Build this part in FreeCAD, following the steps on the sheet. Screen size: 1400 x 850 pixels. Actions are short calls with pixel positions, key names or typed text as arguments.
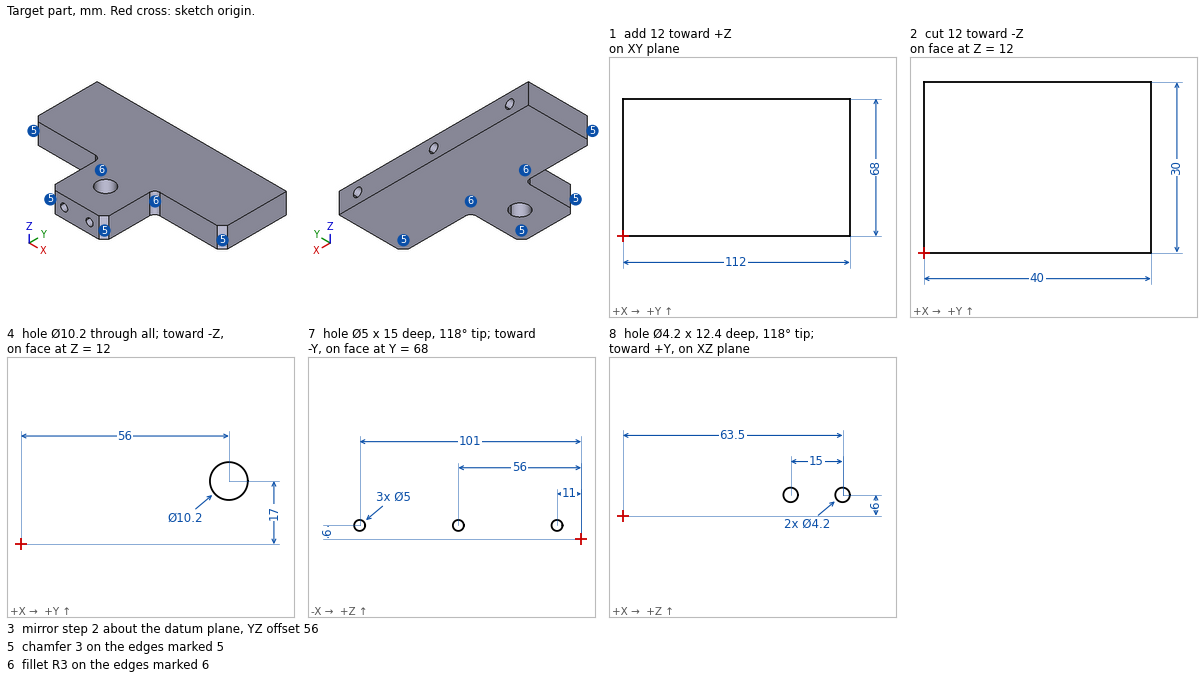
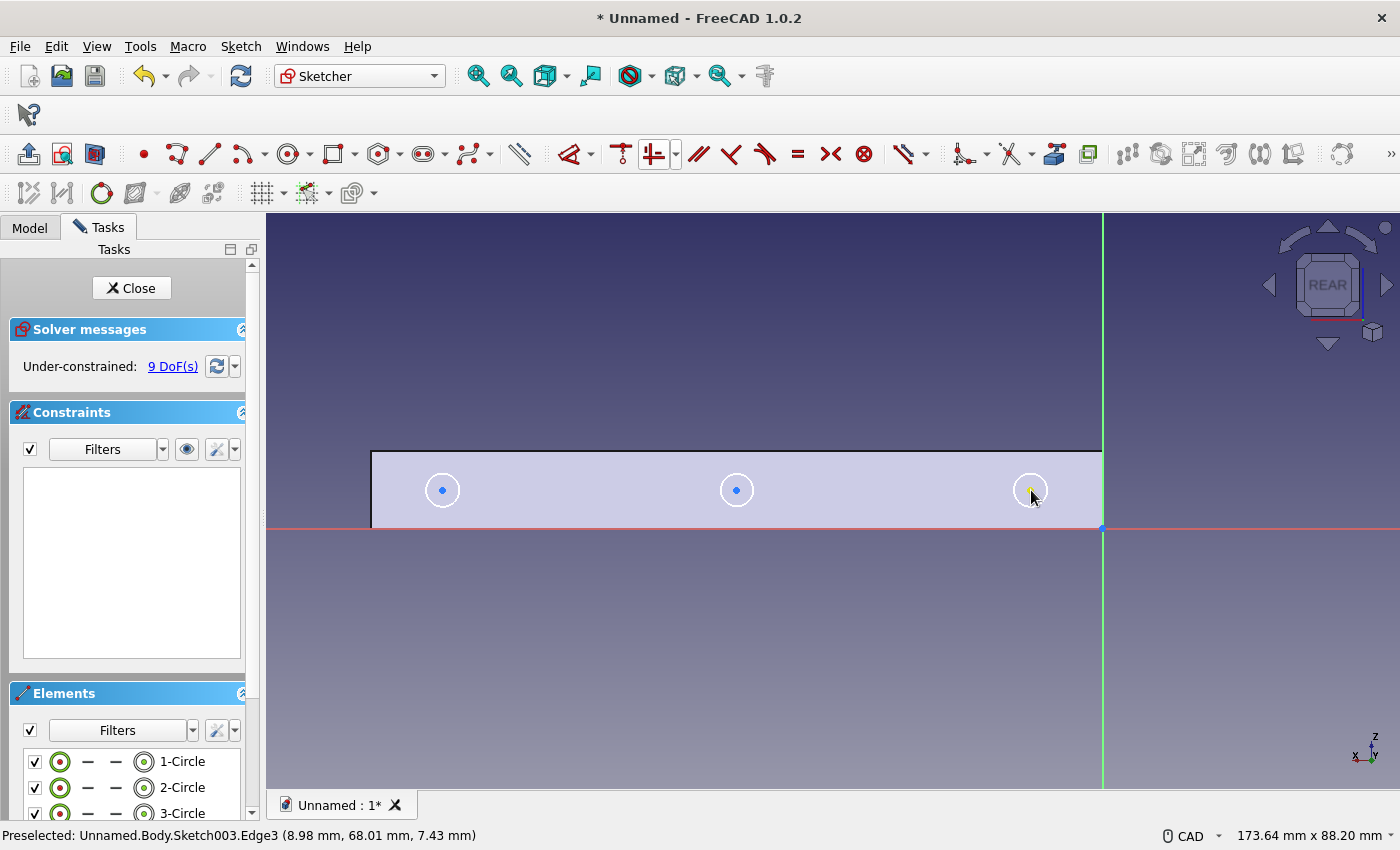
click(454, 478)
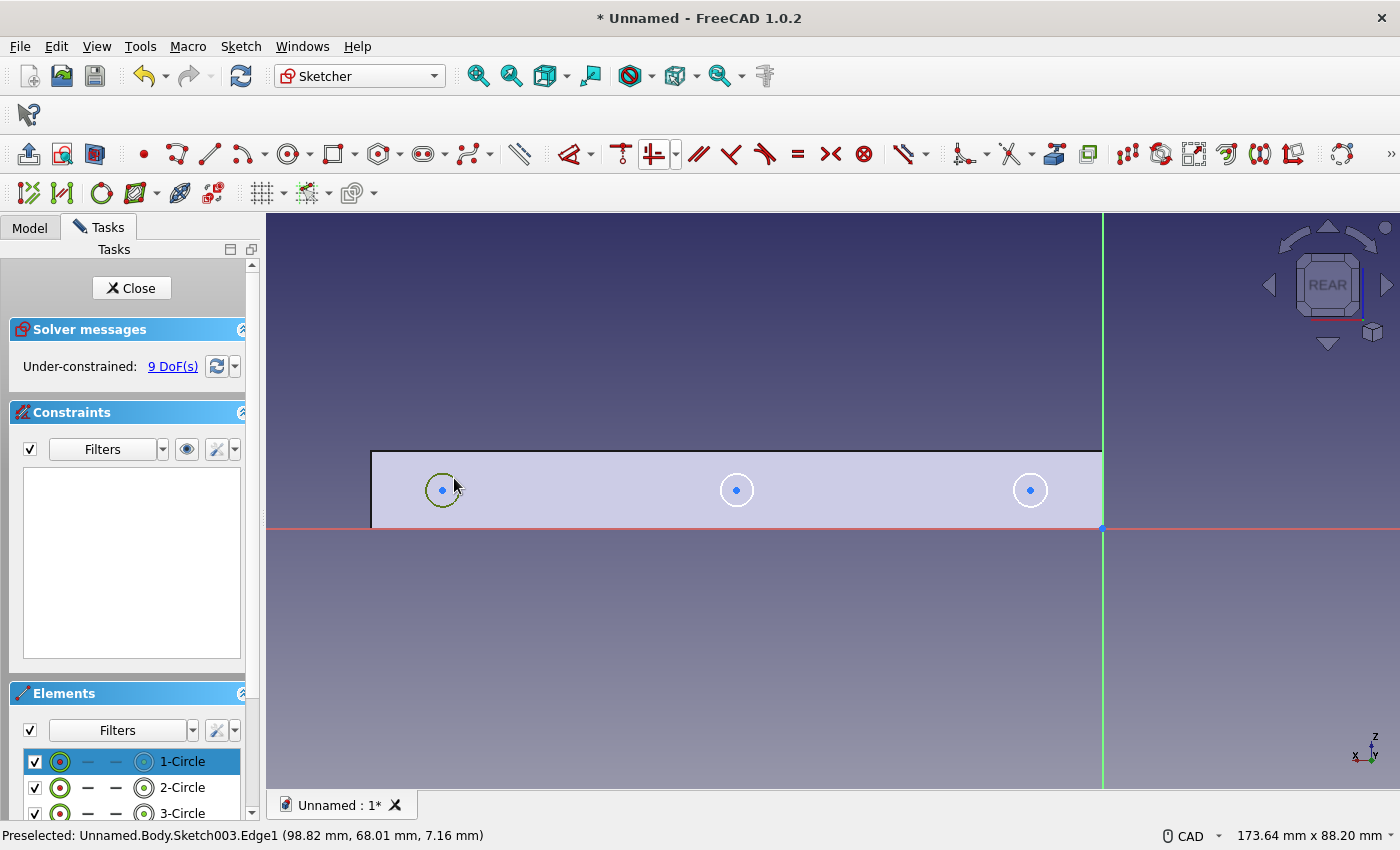
click(748, 479)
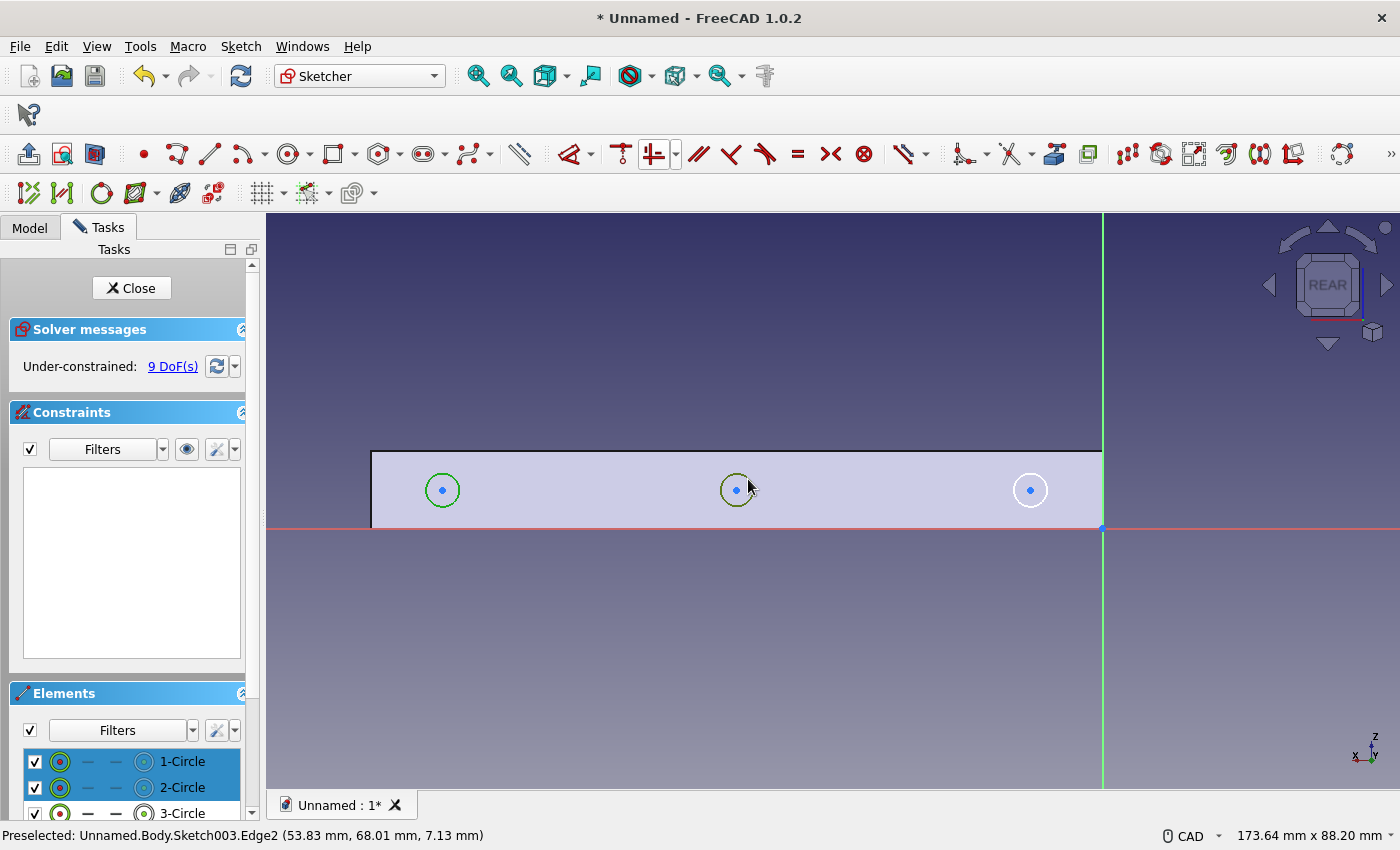
click(1042, 478)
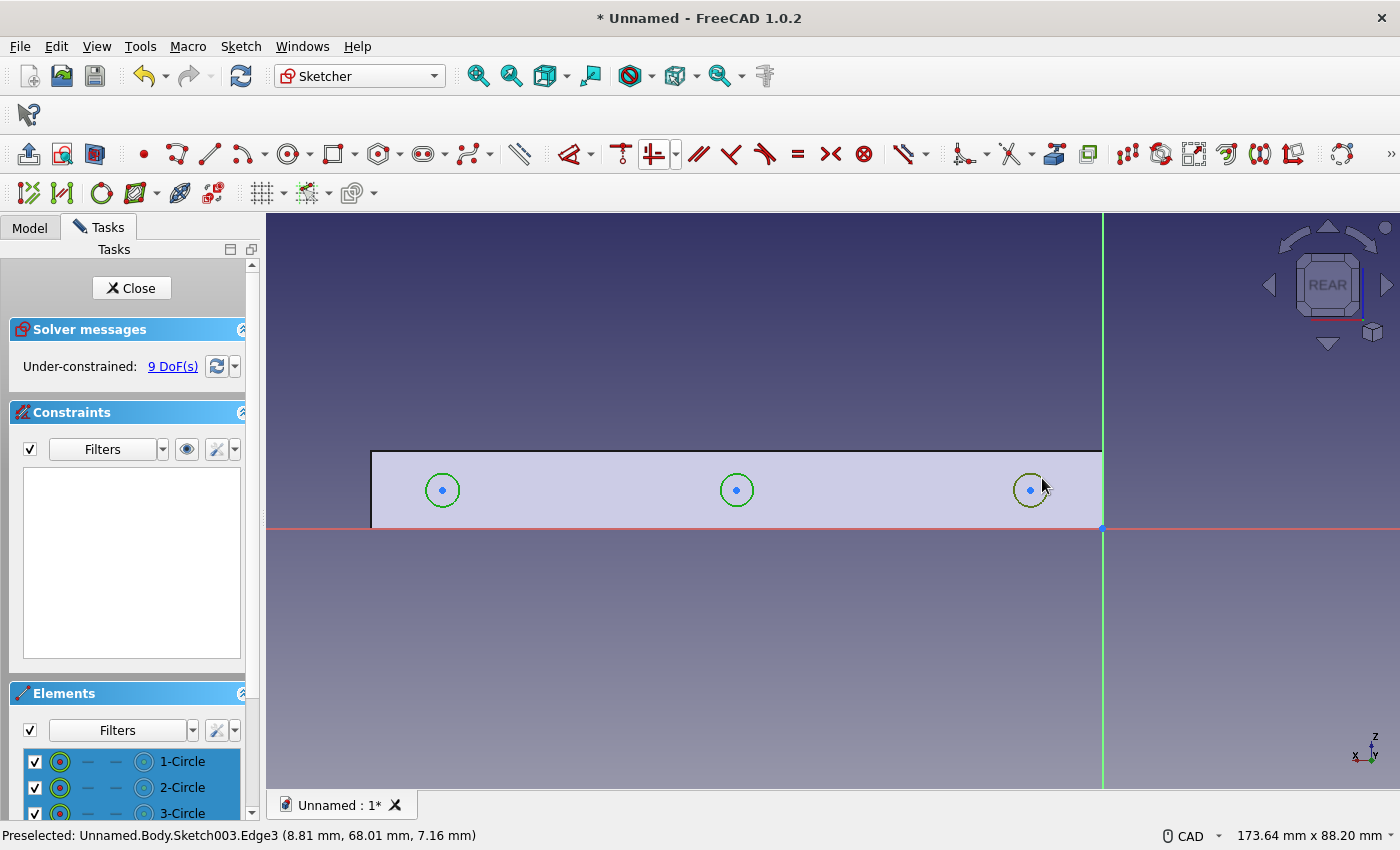
click(798, 154)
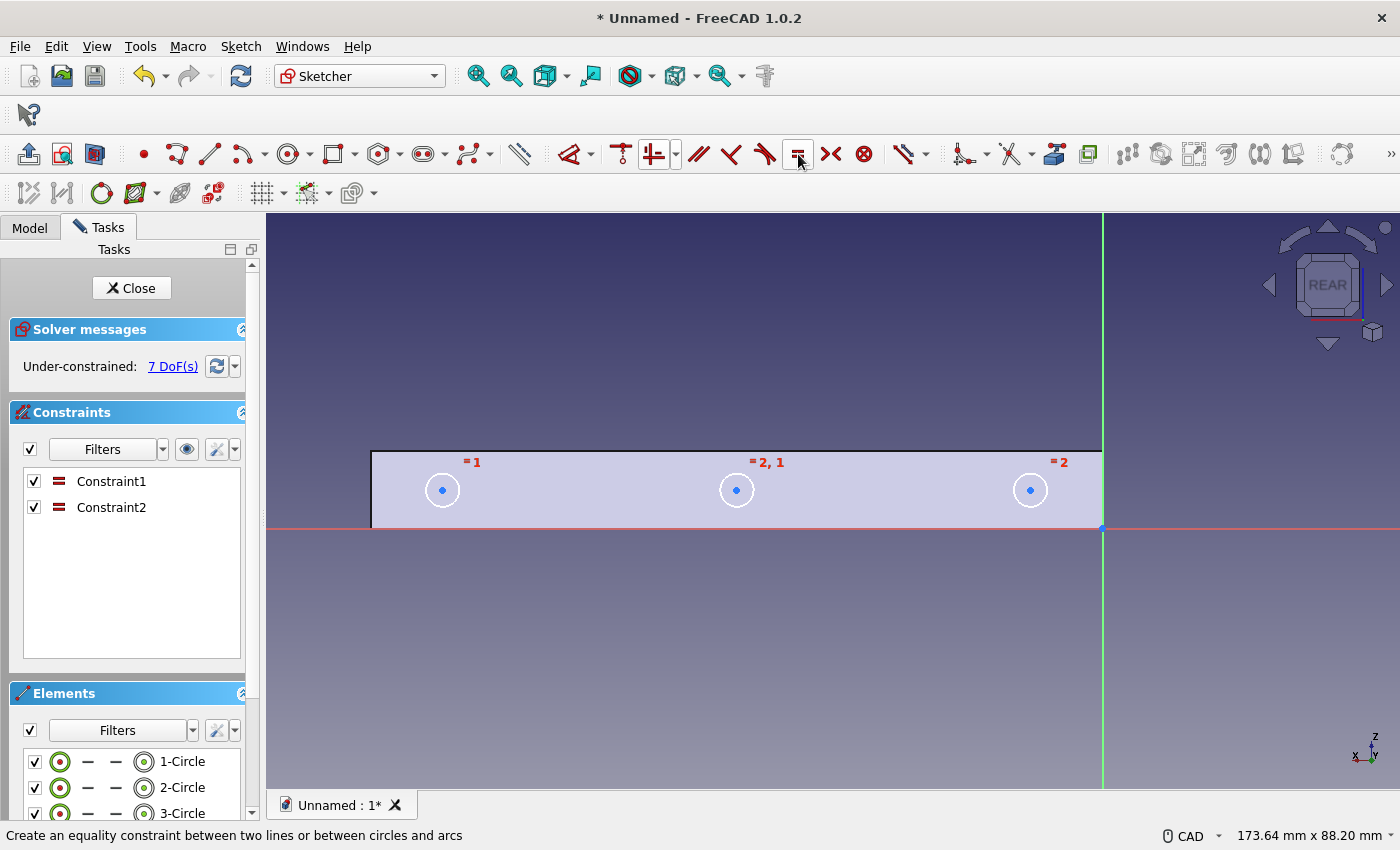
click(443, 490)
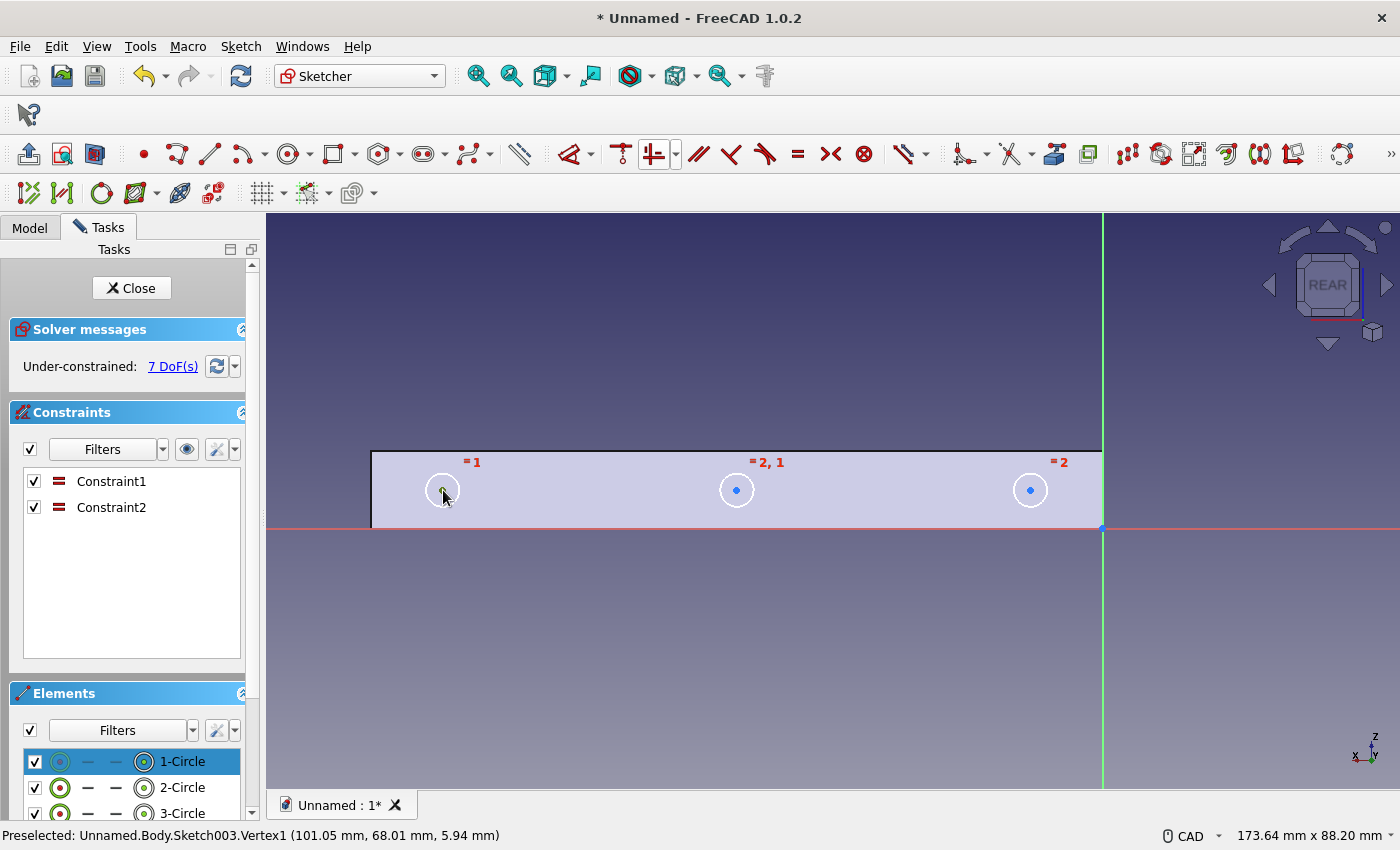
click(737, 490)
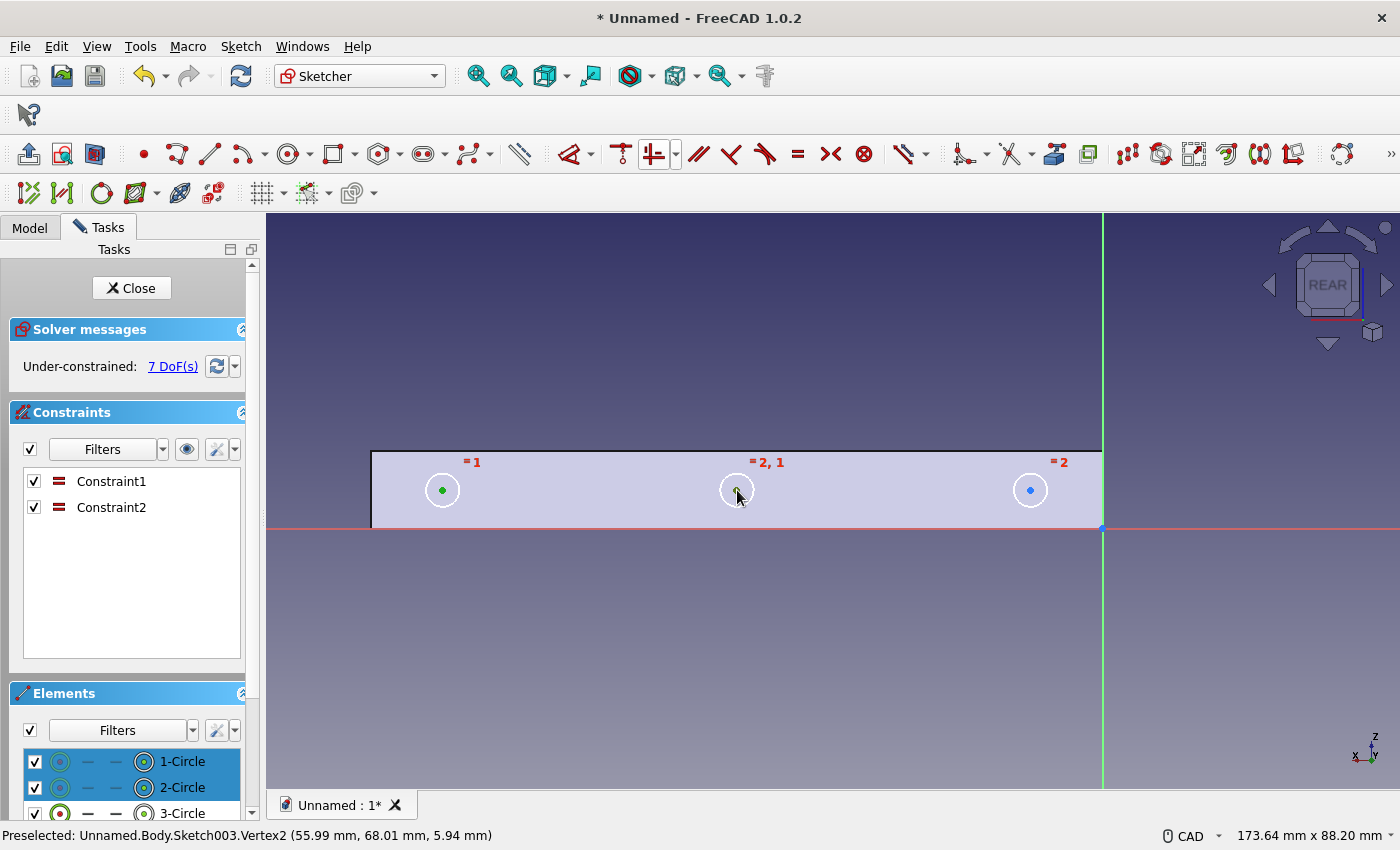
click(676, 154)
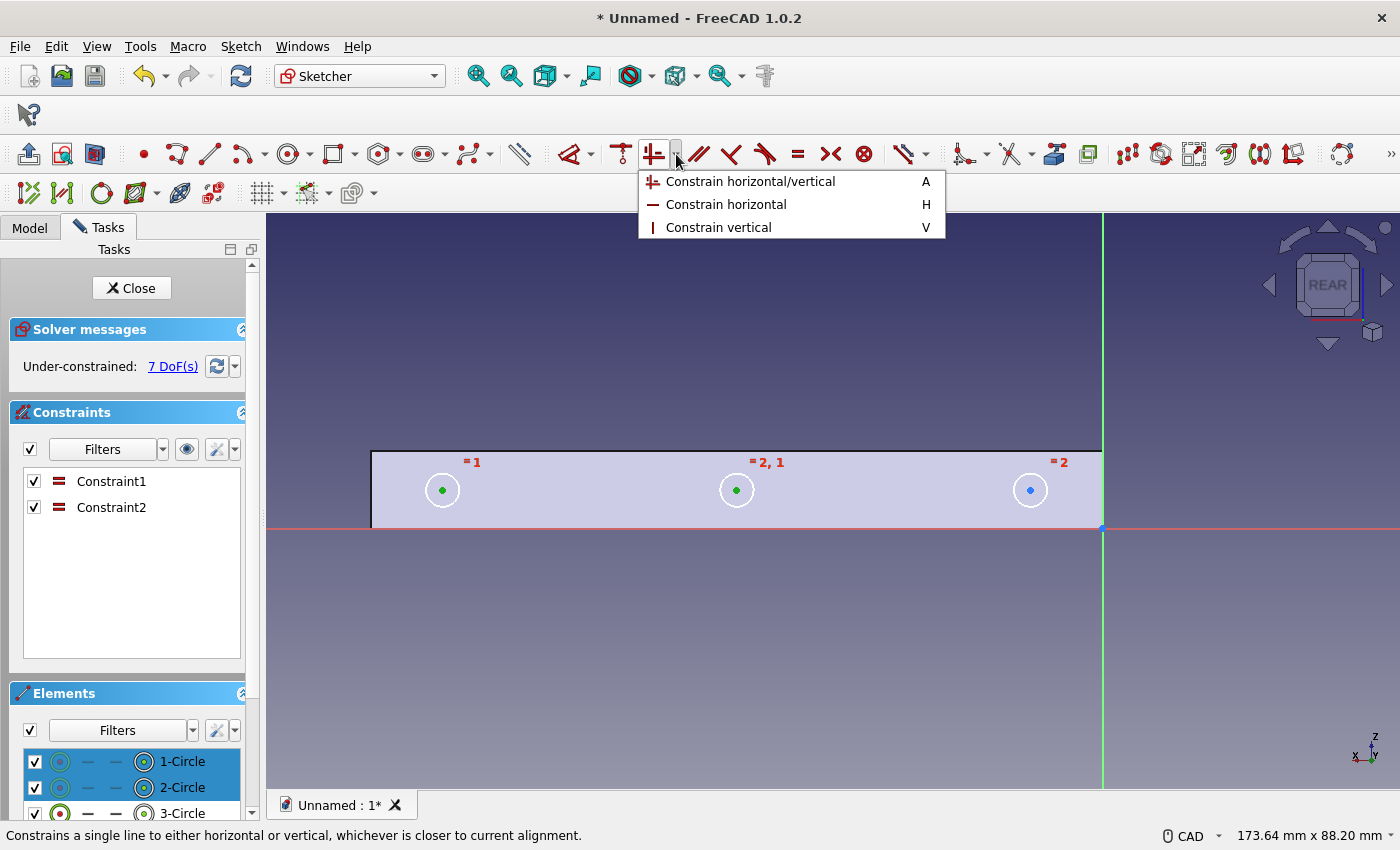
click(792, 204)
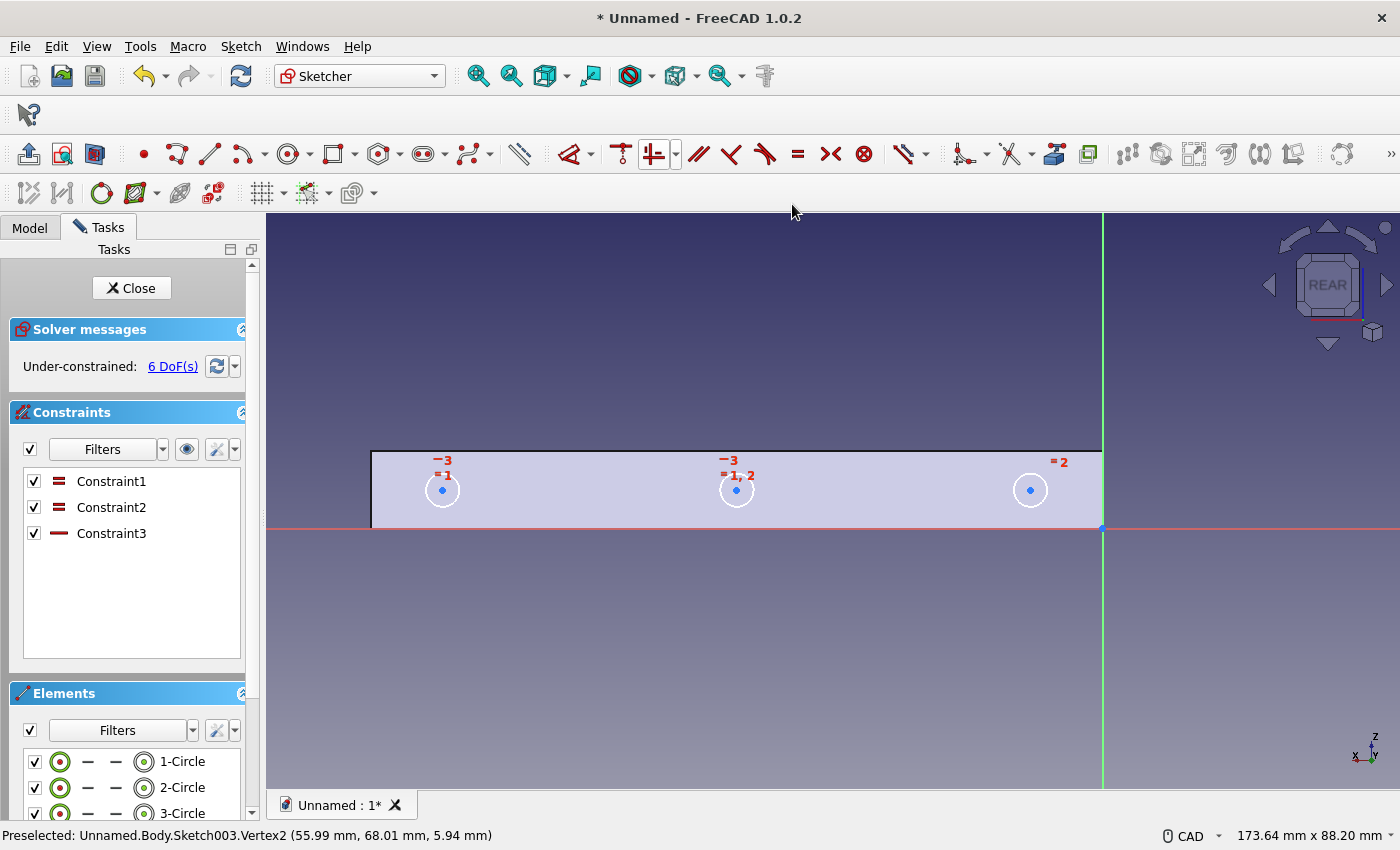
click(737, 490)